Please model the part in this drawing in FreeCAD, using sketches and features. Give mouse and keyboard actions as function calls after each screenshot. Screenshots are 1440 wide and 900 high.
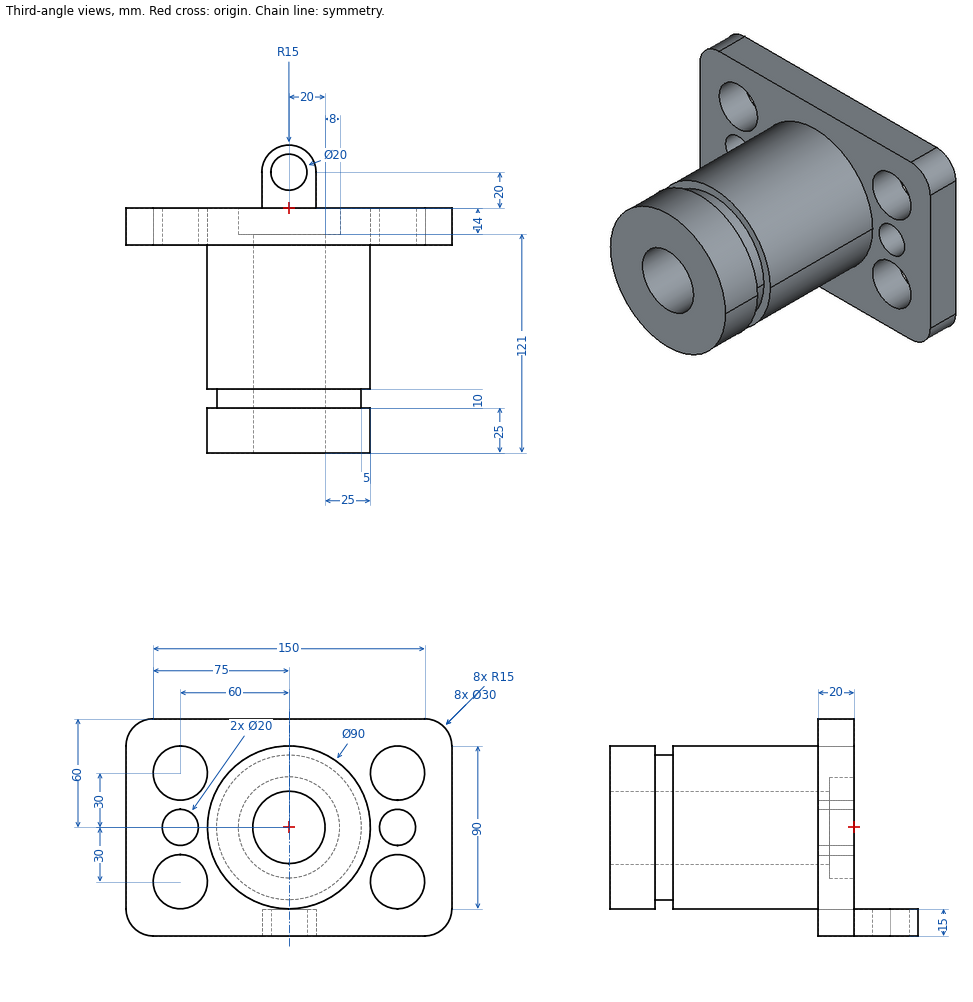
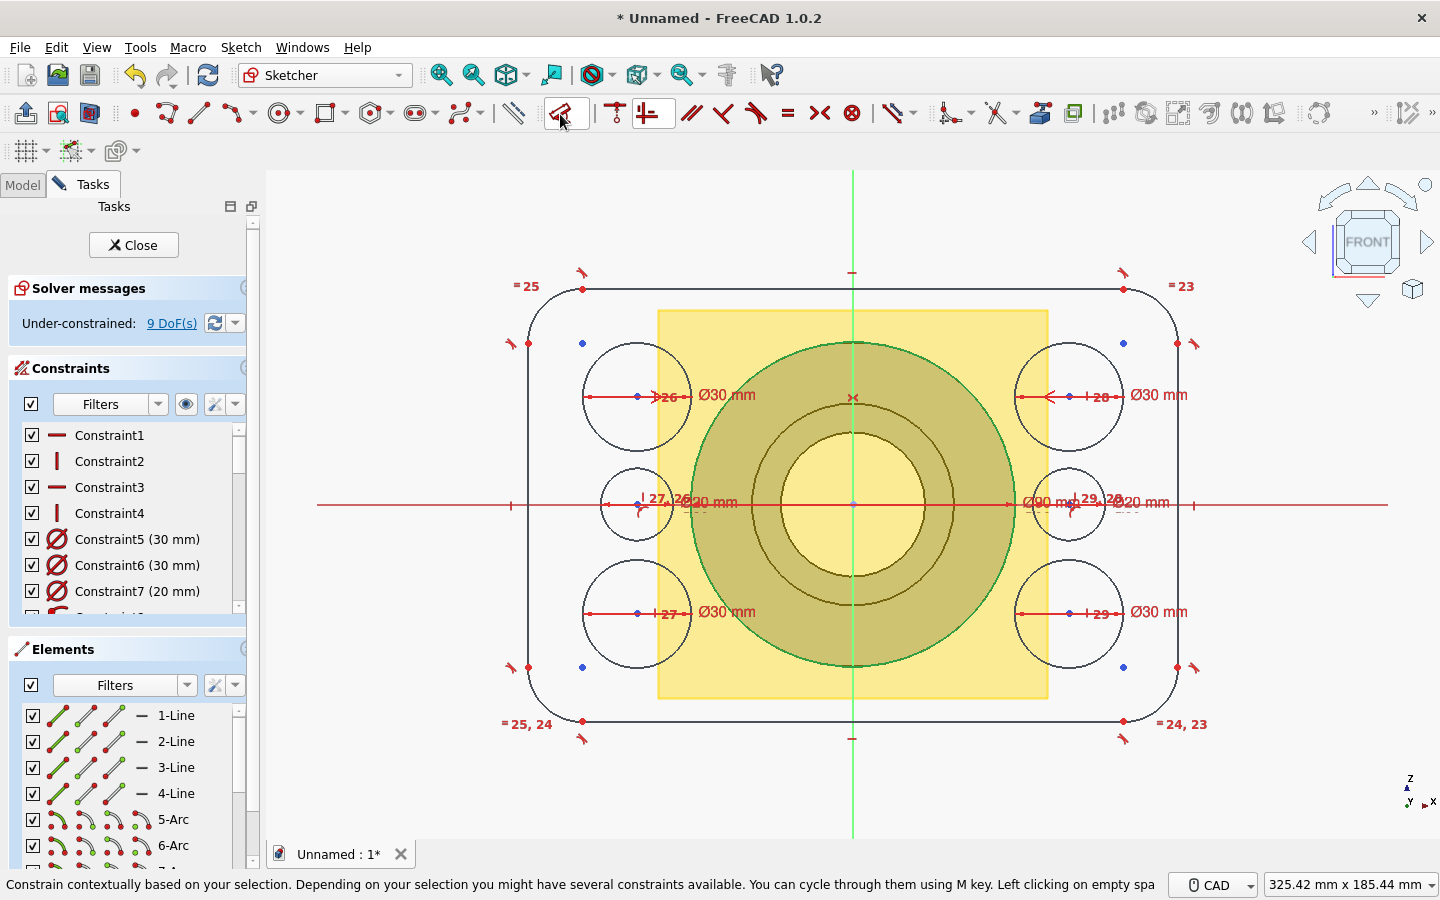
click(1172, 319)
click(1201, 305)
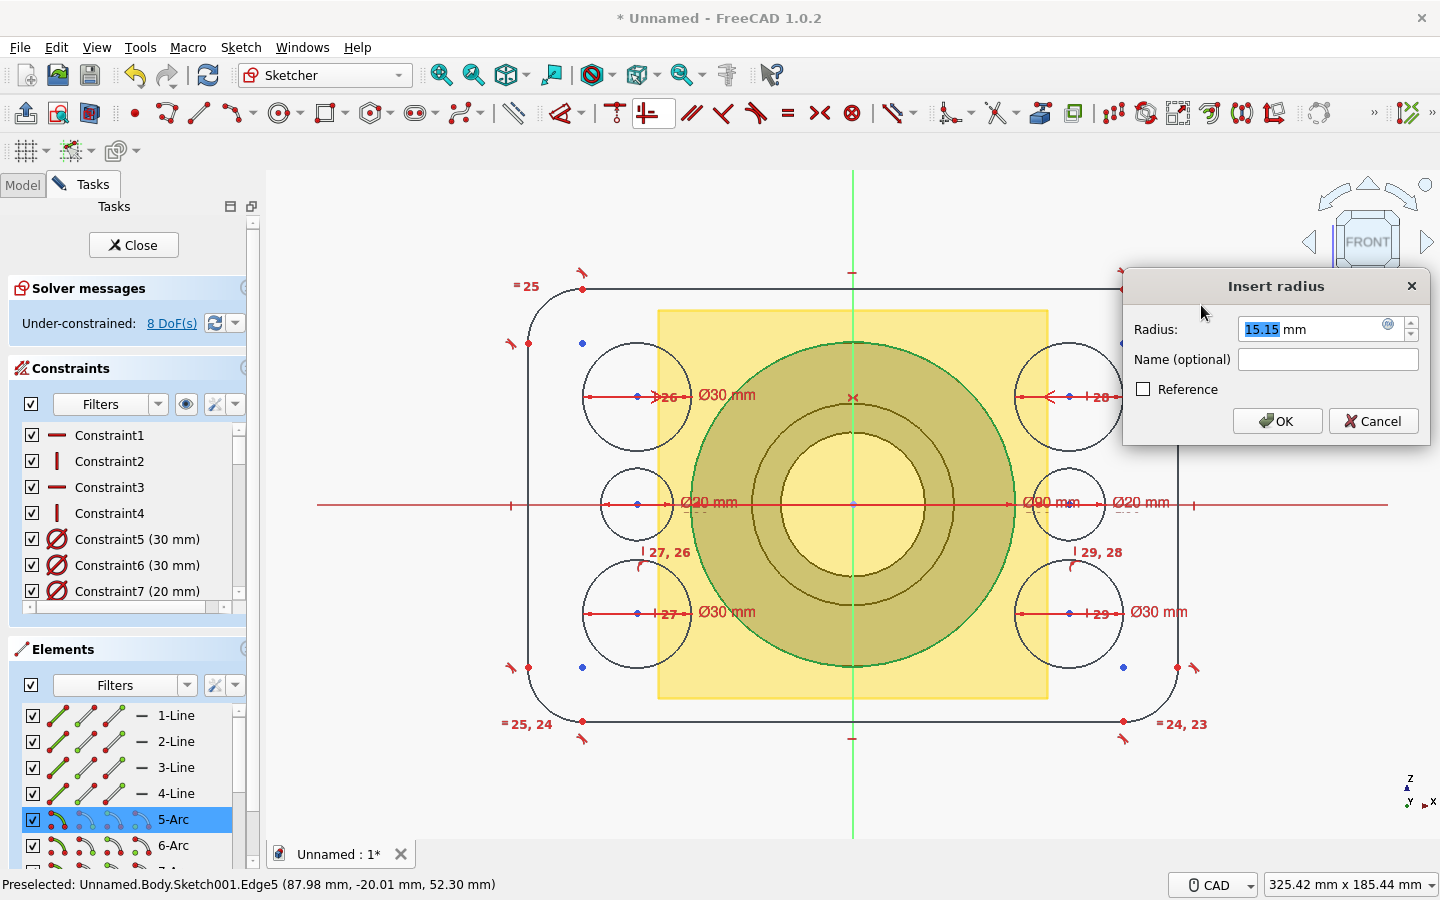
text(15)
key(Return)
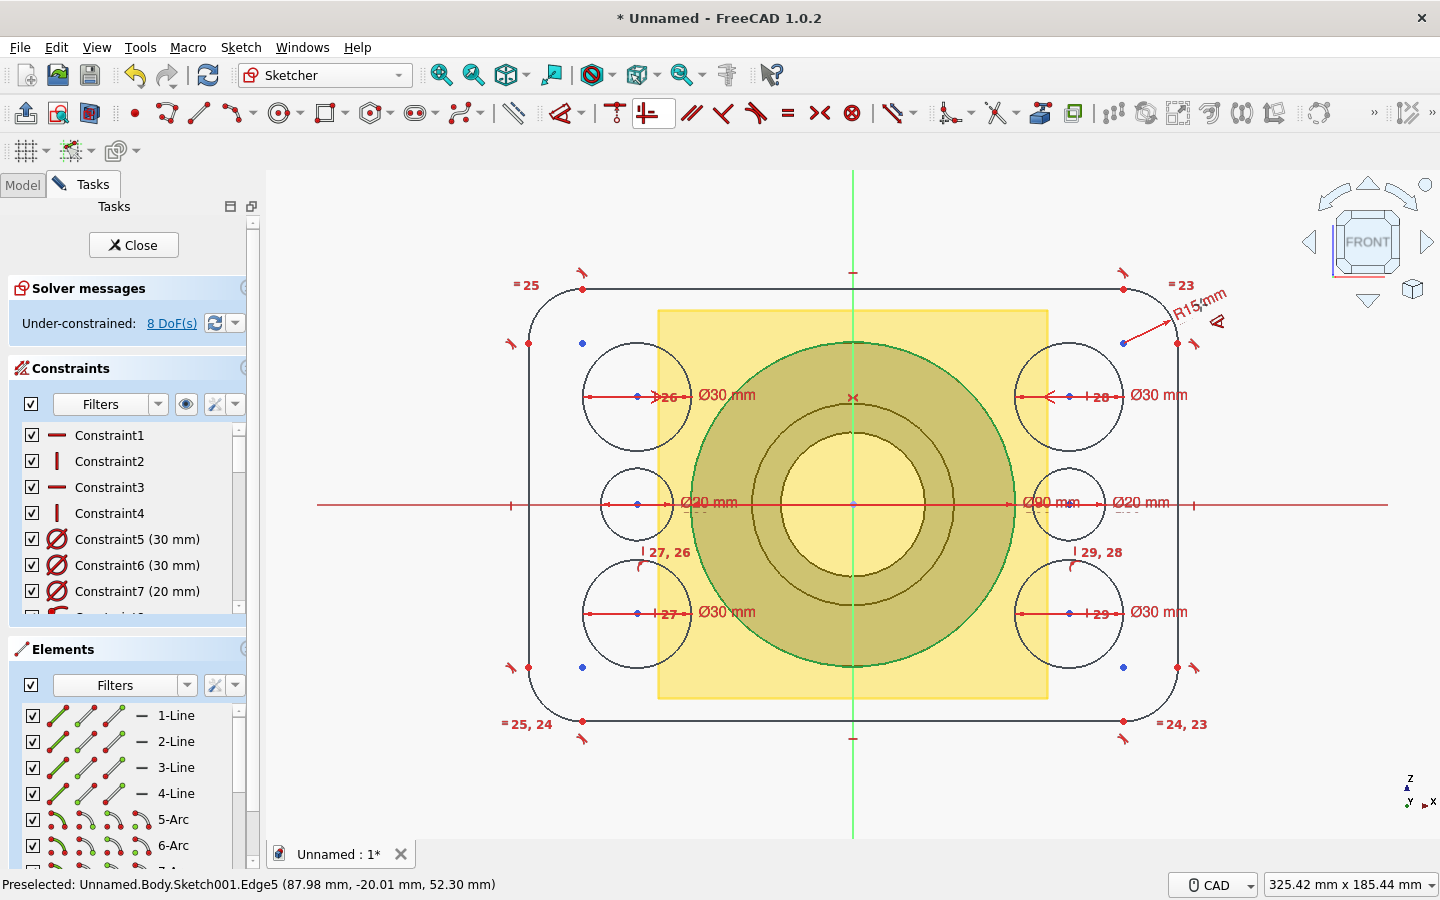
click(1178, 440)
click(1212, 431)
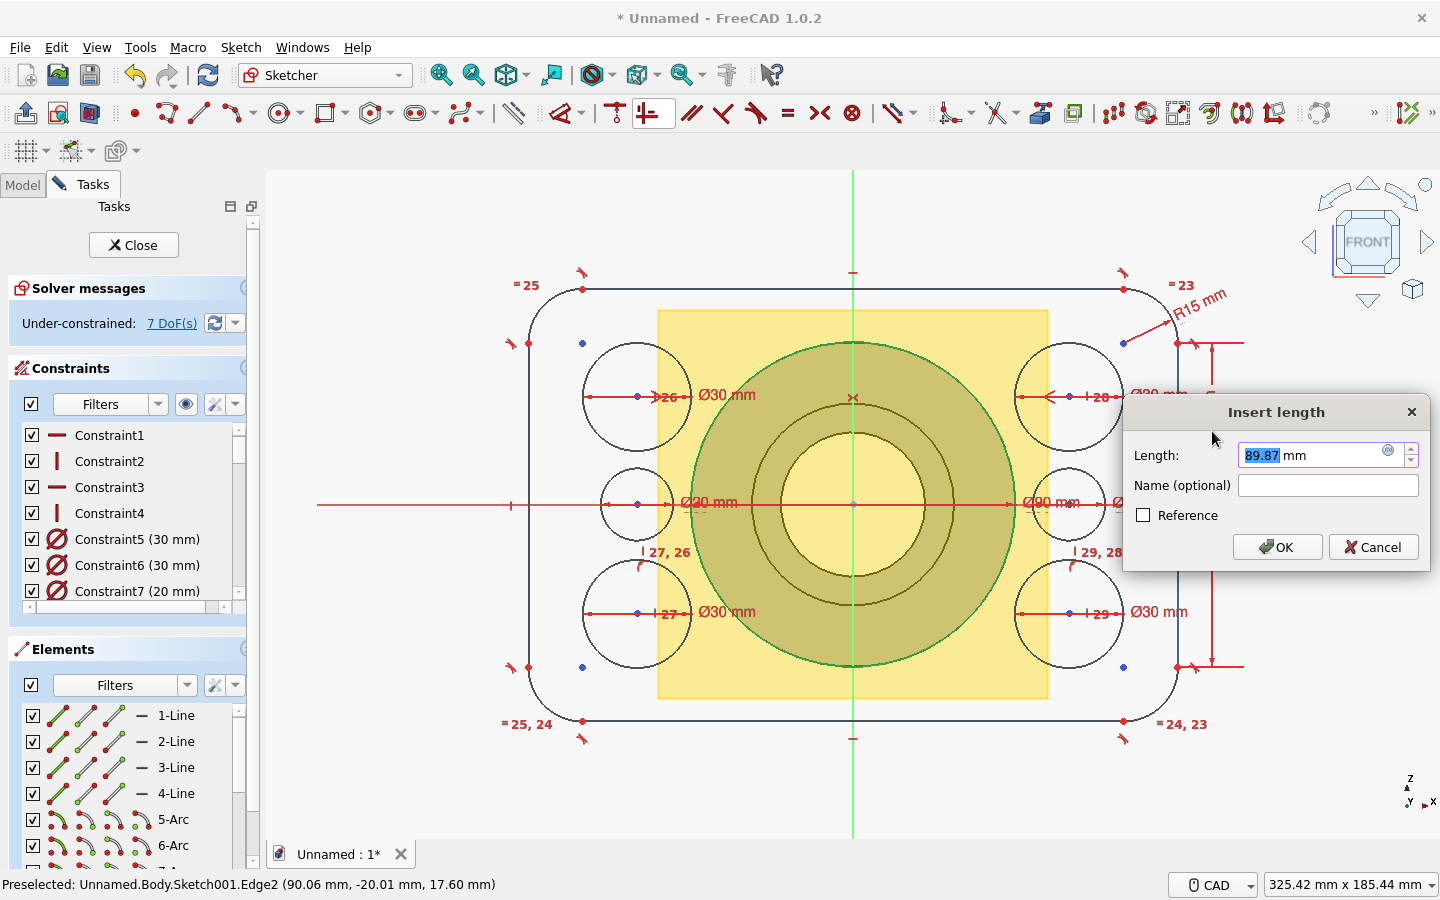
text(90)
key(Return)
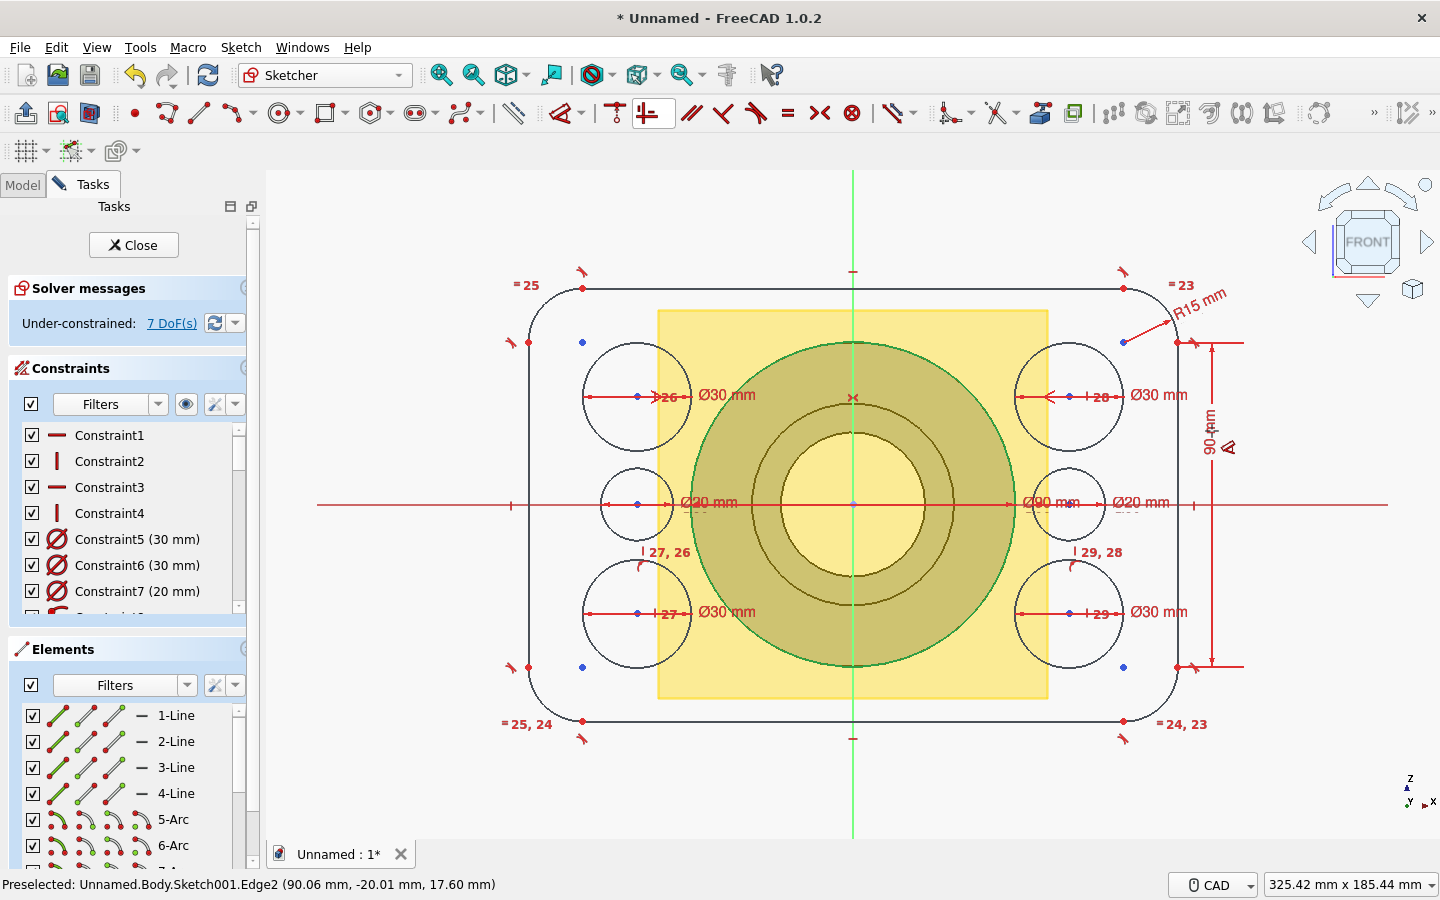
click(637, 397)
click(745, 363)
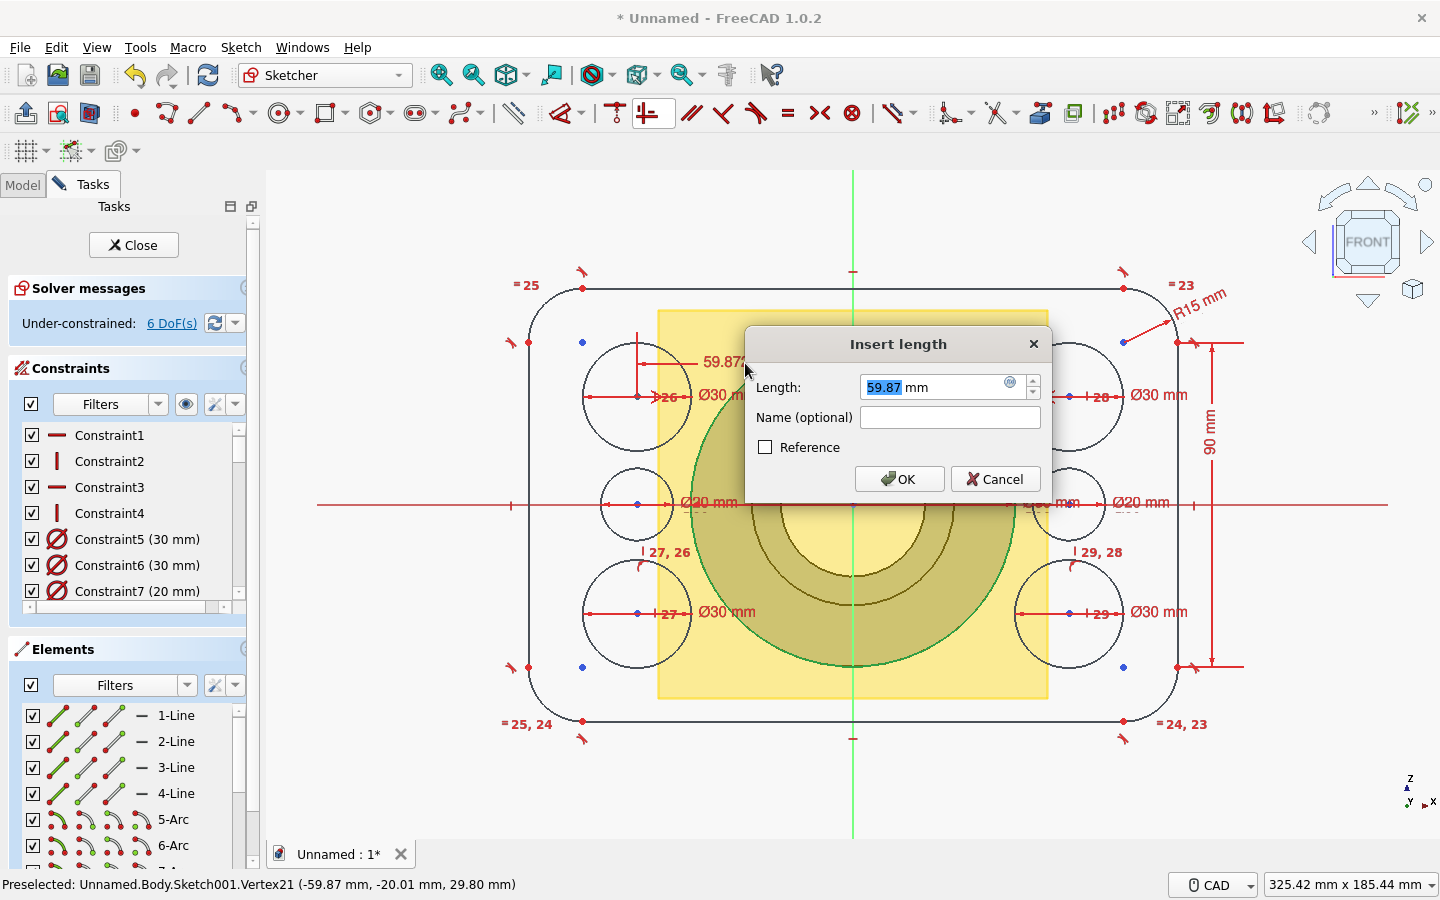
text(60)
key(Return)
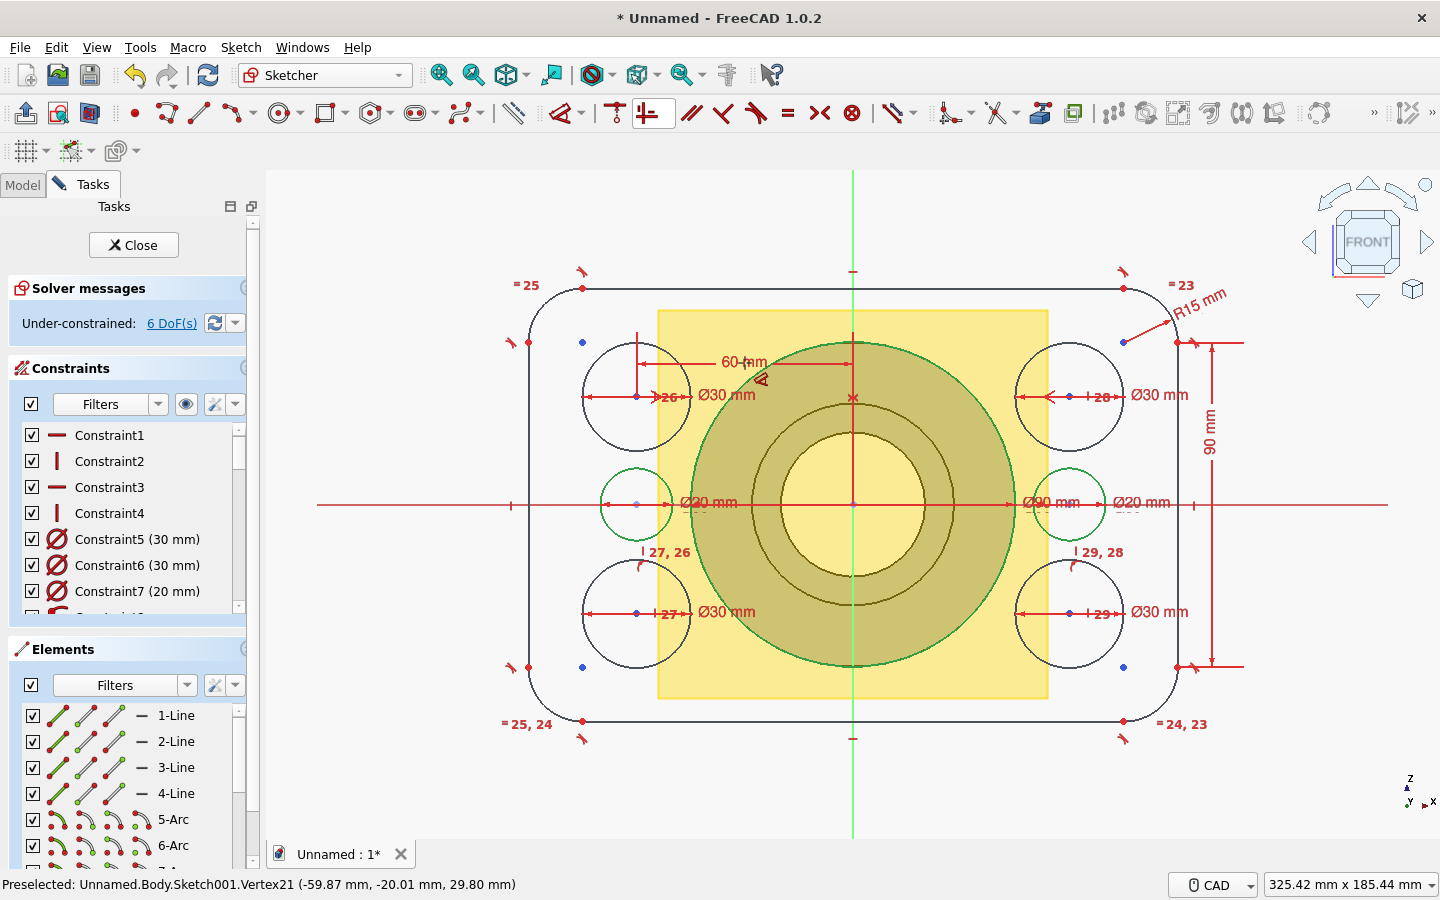
click(637, 397)
click(603, 413)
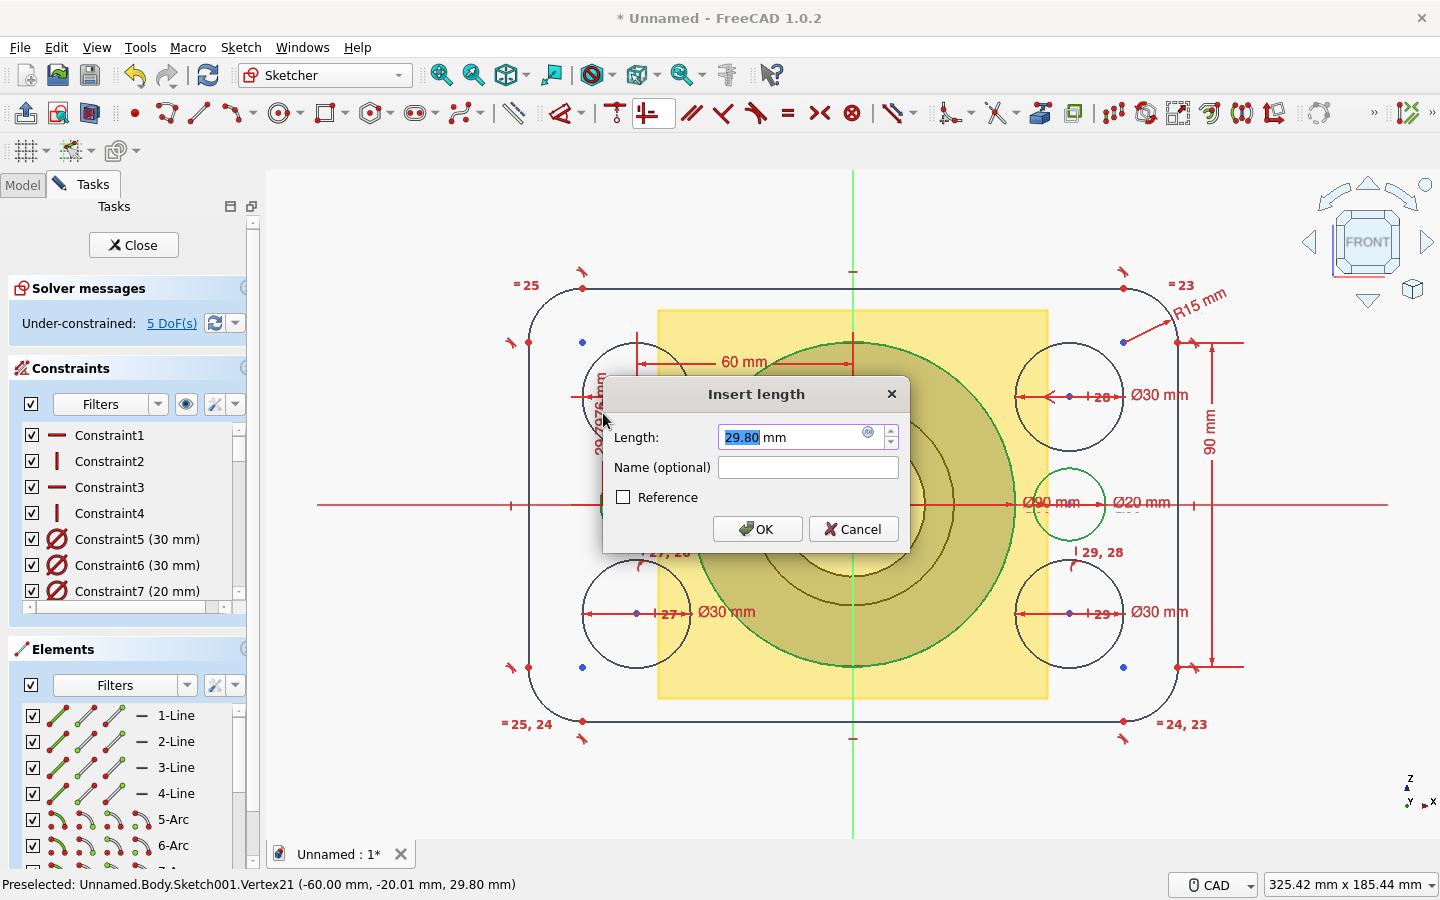
text(30)
key(Return)